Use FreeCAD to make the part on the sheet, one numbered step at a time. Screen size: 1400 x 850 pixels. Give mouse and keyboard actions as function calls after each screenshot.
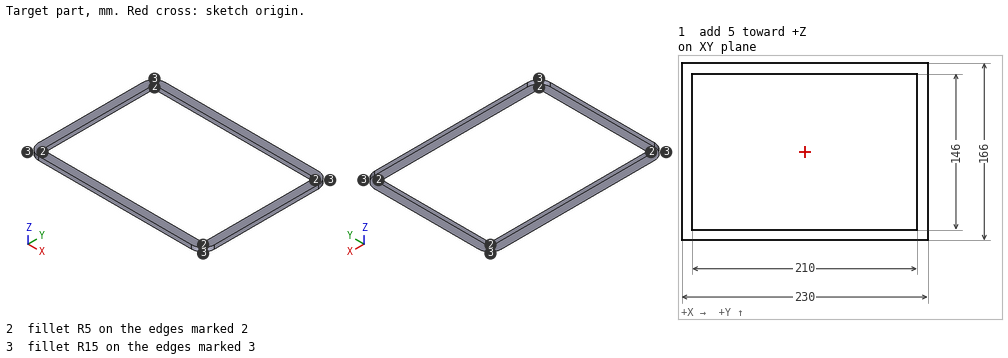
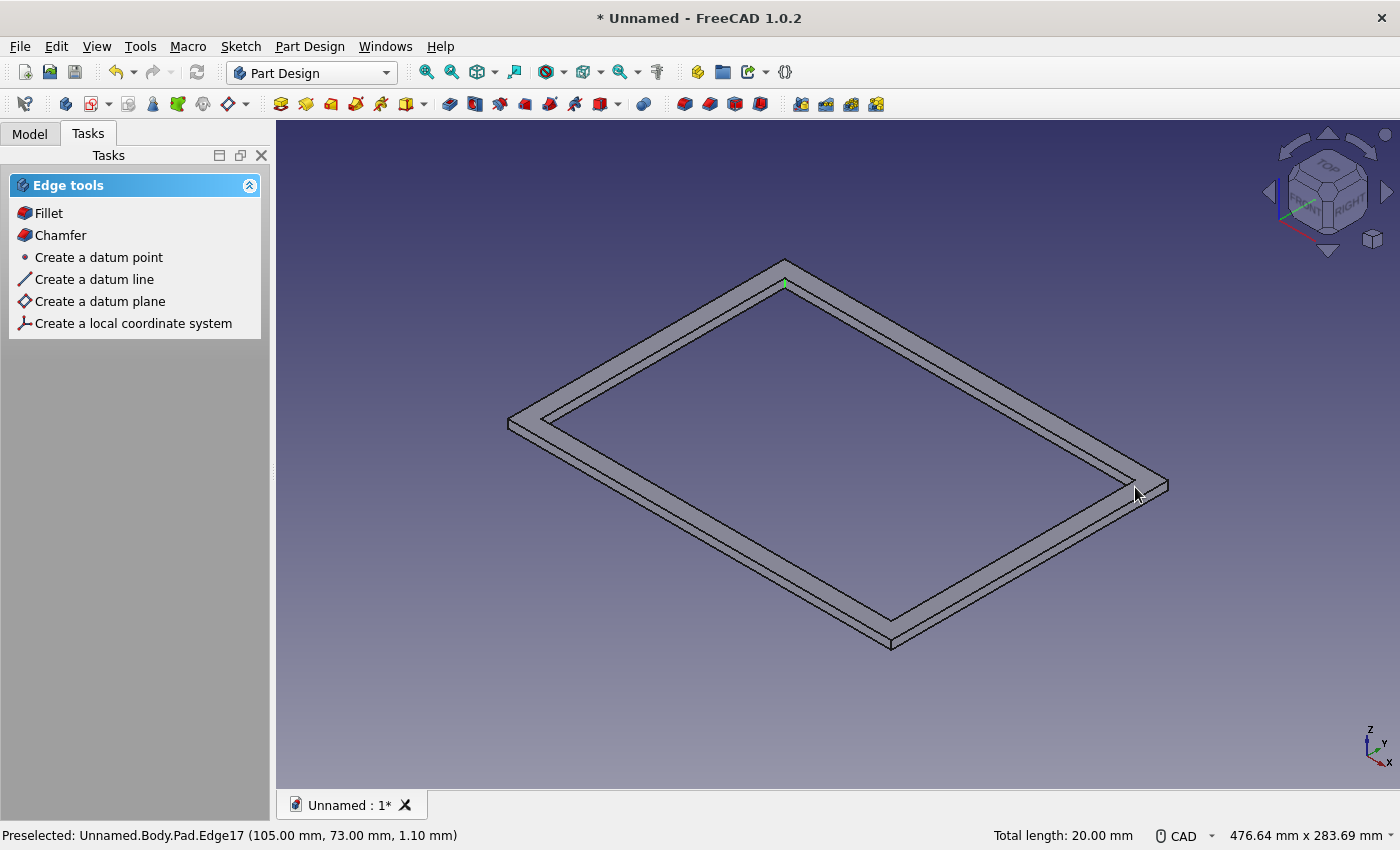
click(685, 104)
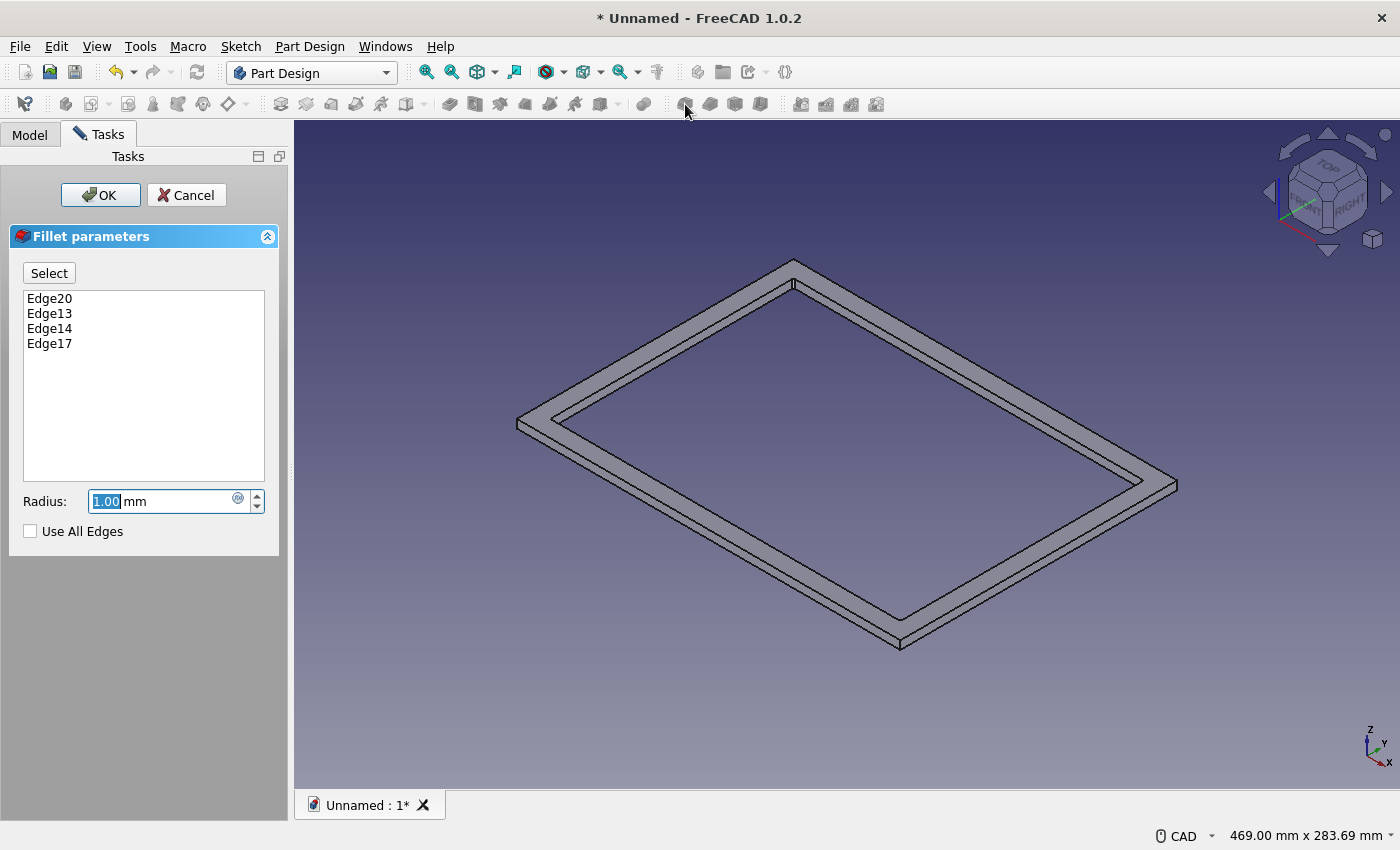
text(5)
key(Tab)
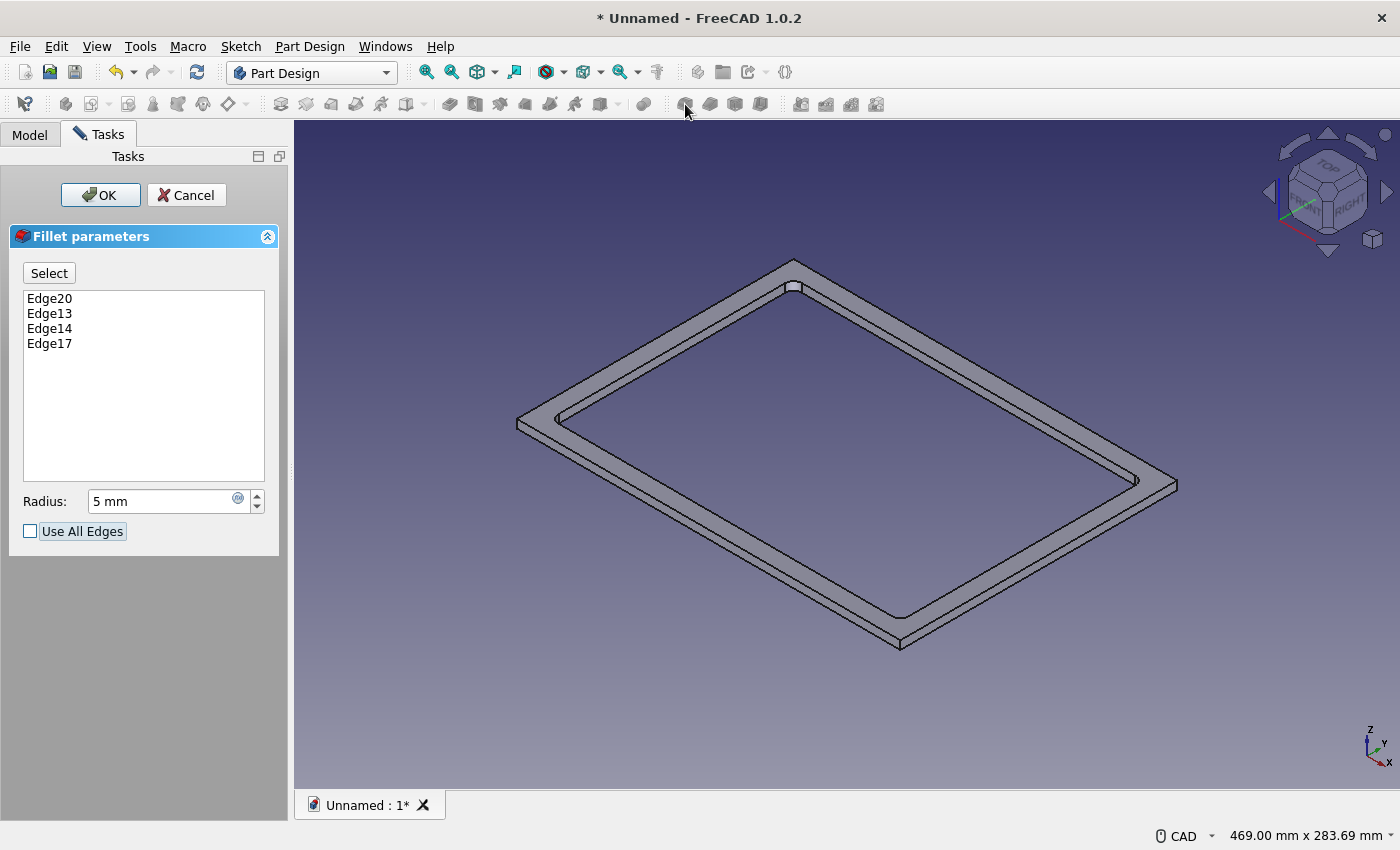
click(101, 195)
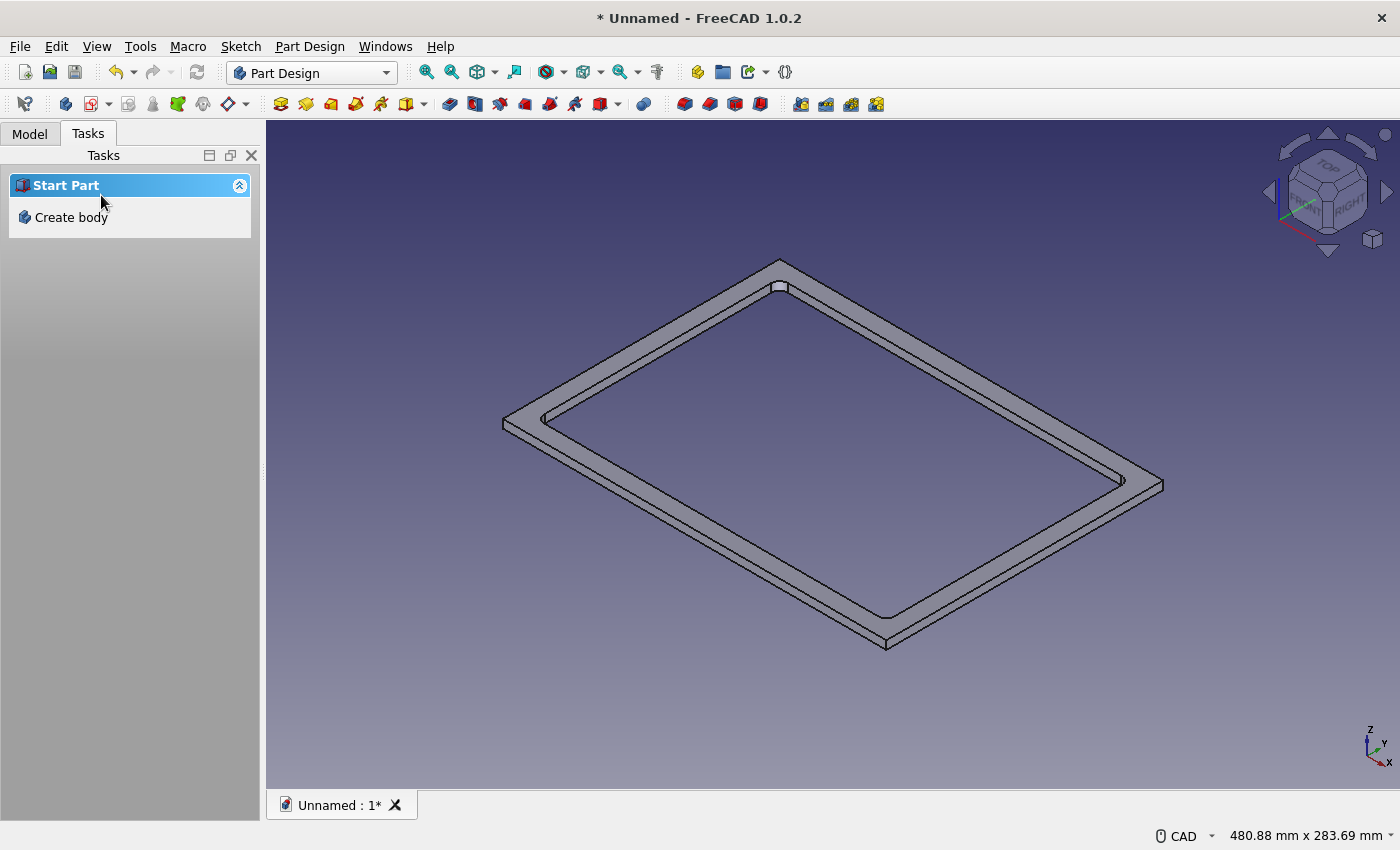
click(886, 646)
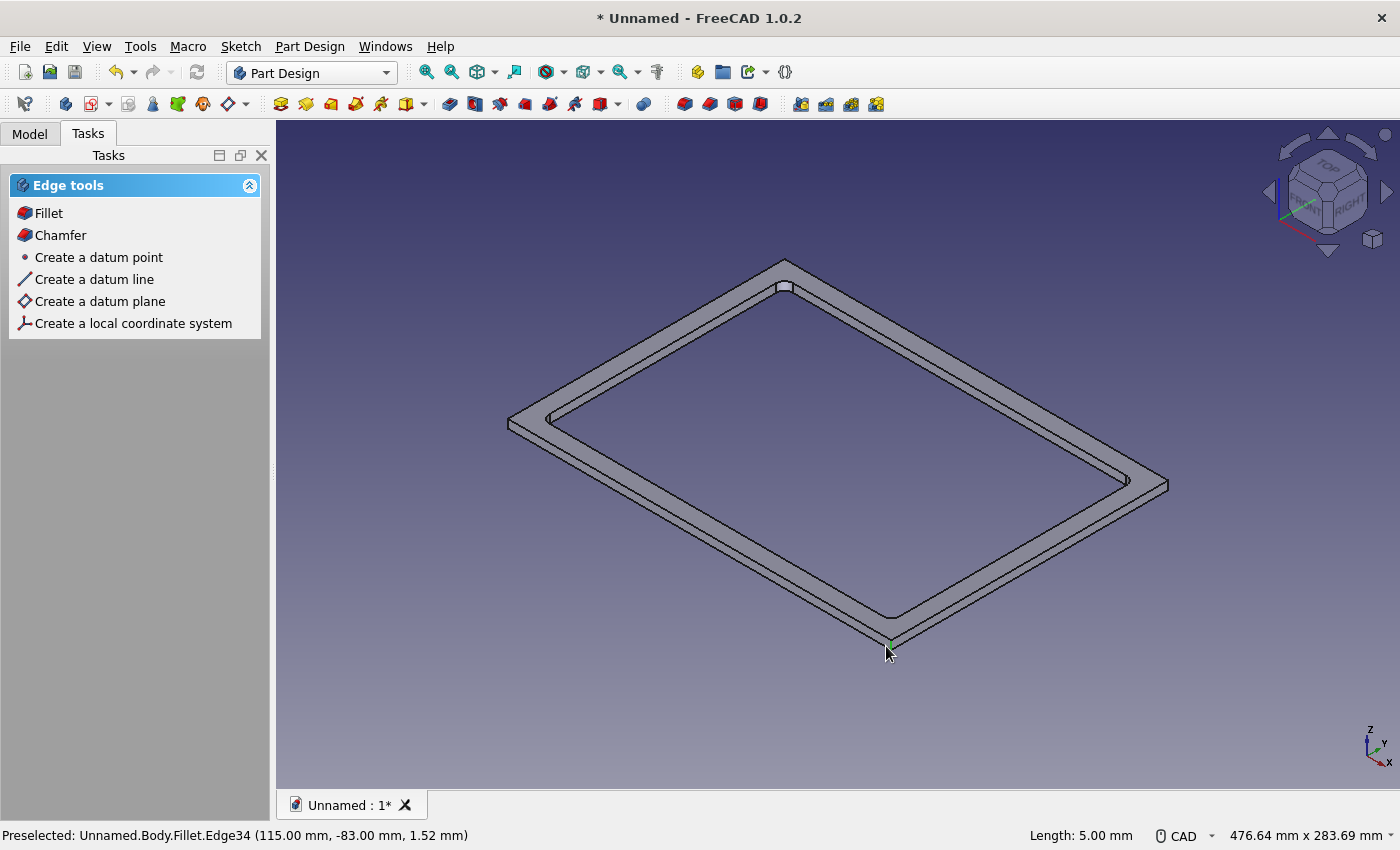
scroll(785, 263, up, 7)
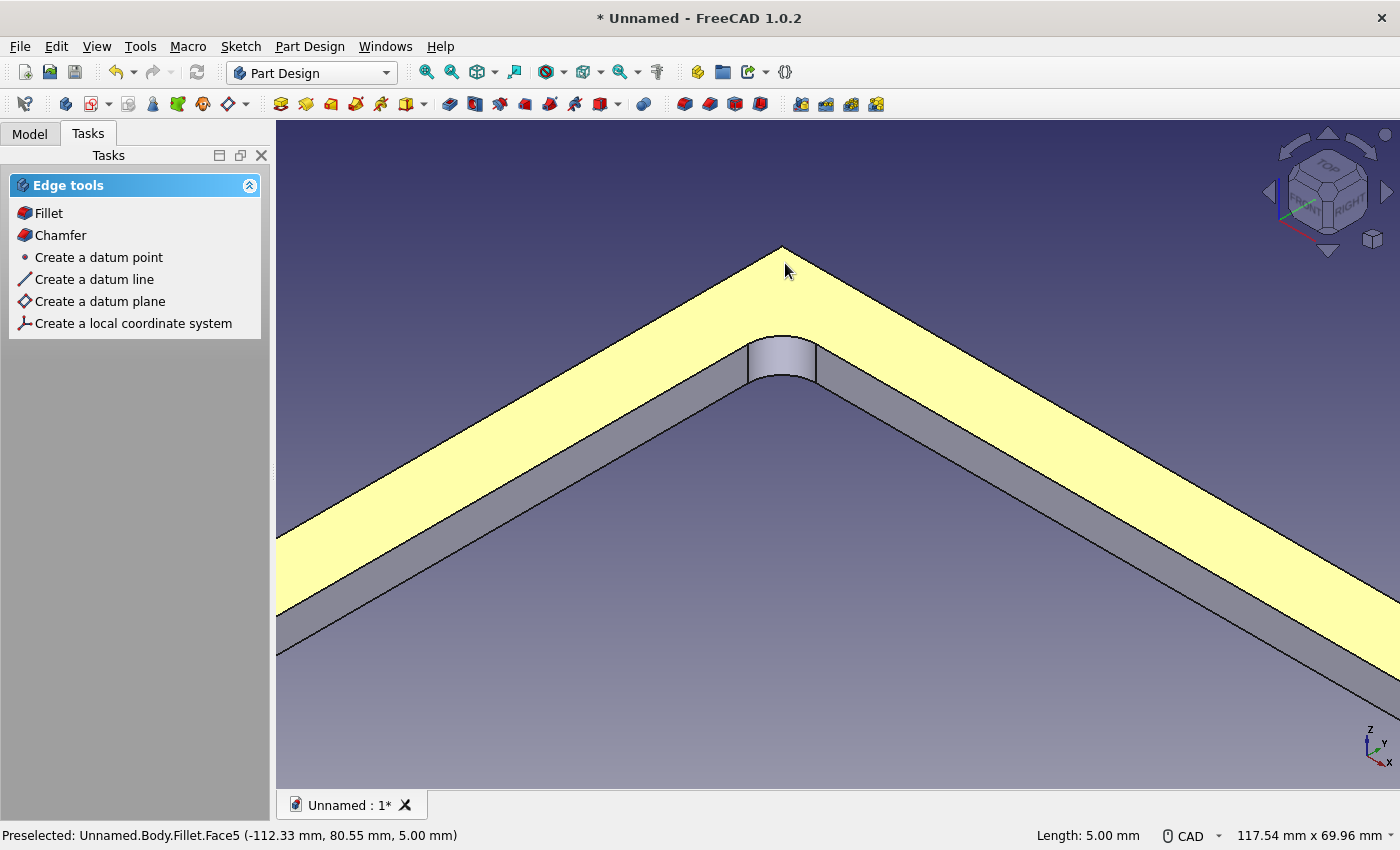
key(v)
key(f)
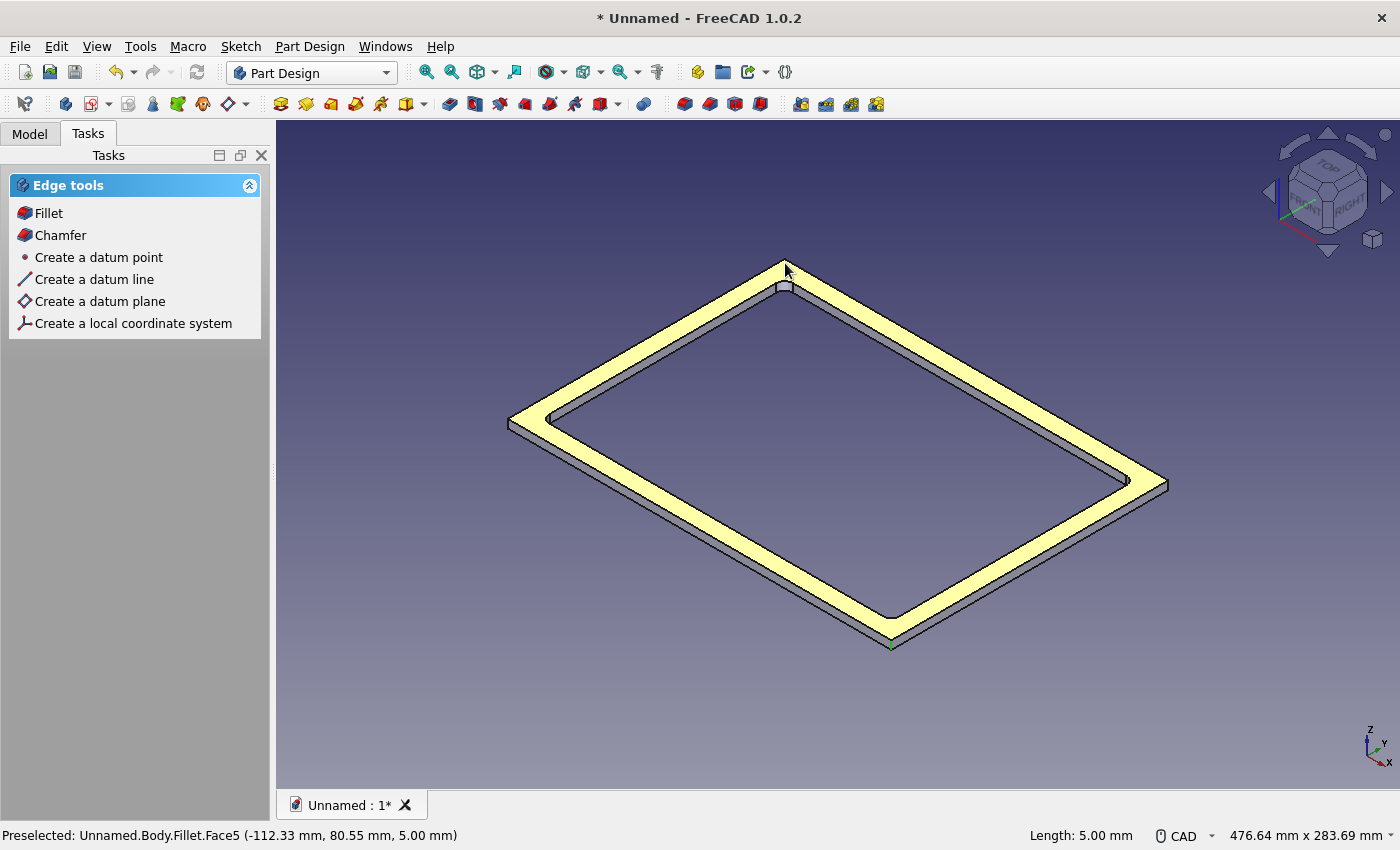
key(2)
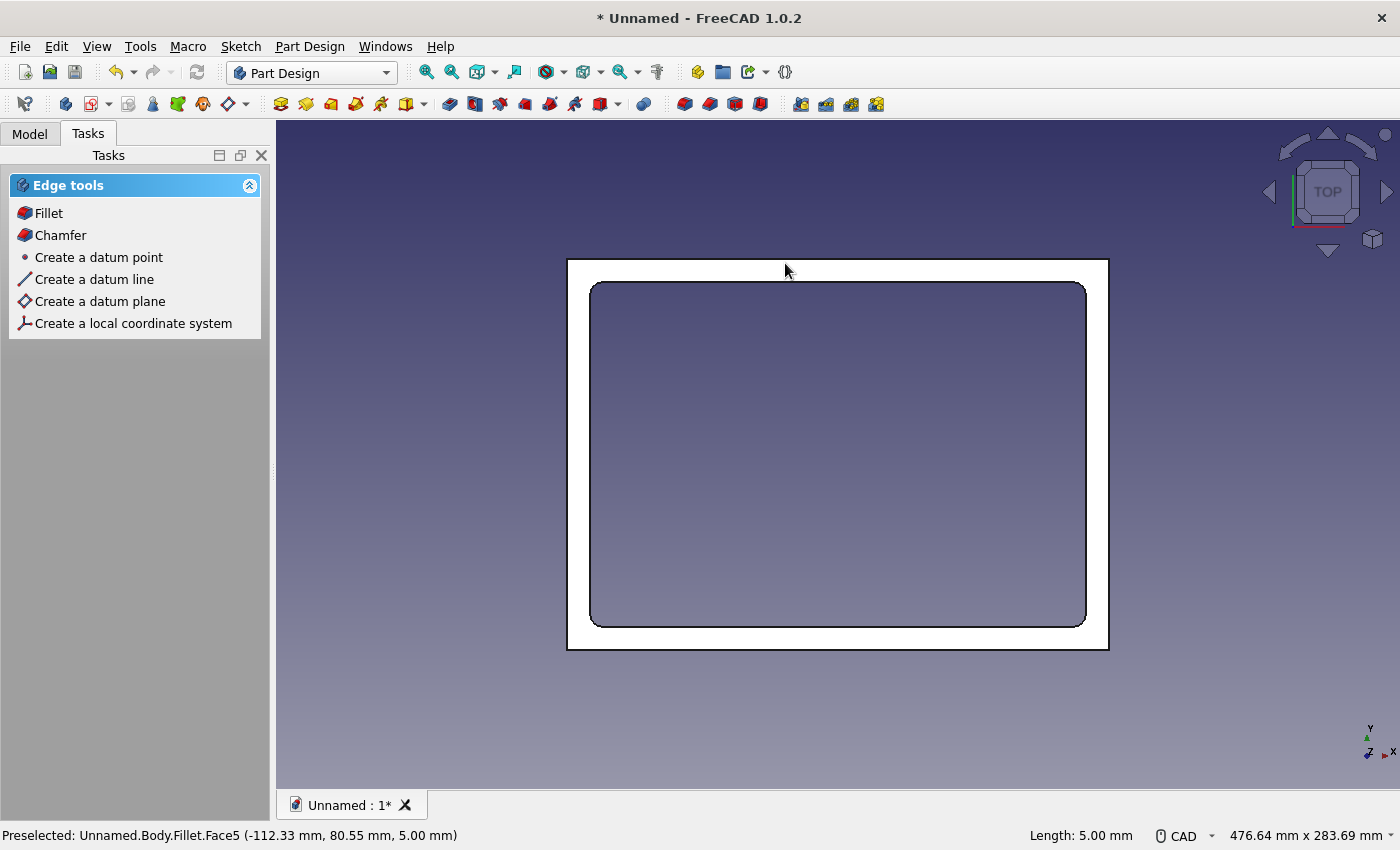
scroll(567, 258, up, 7)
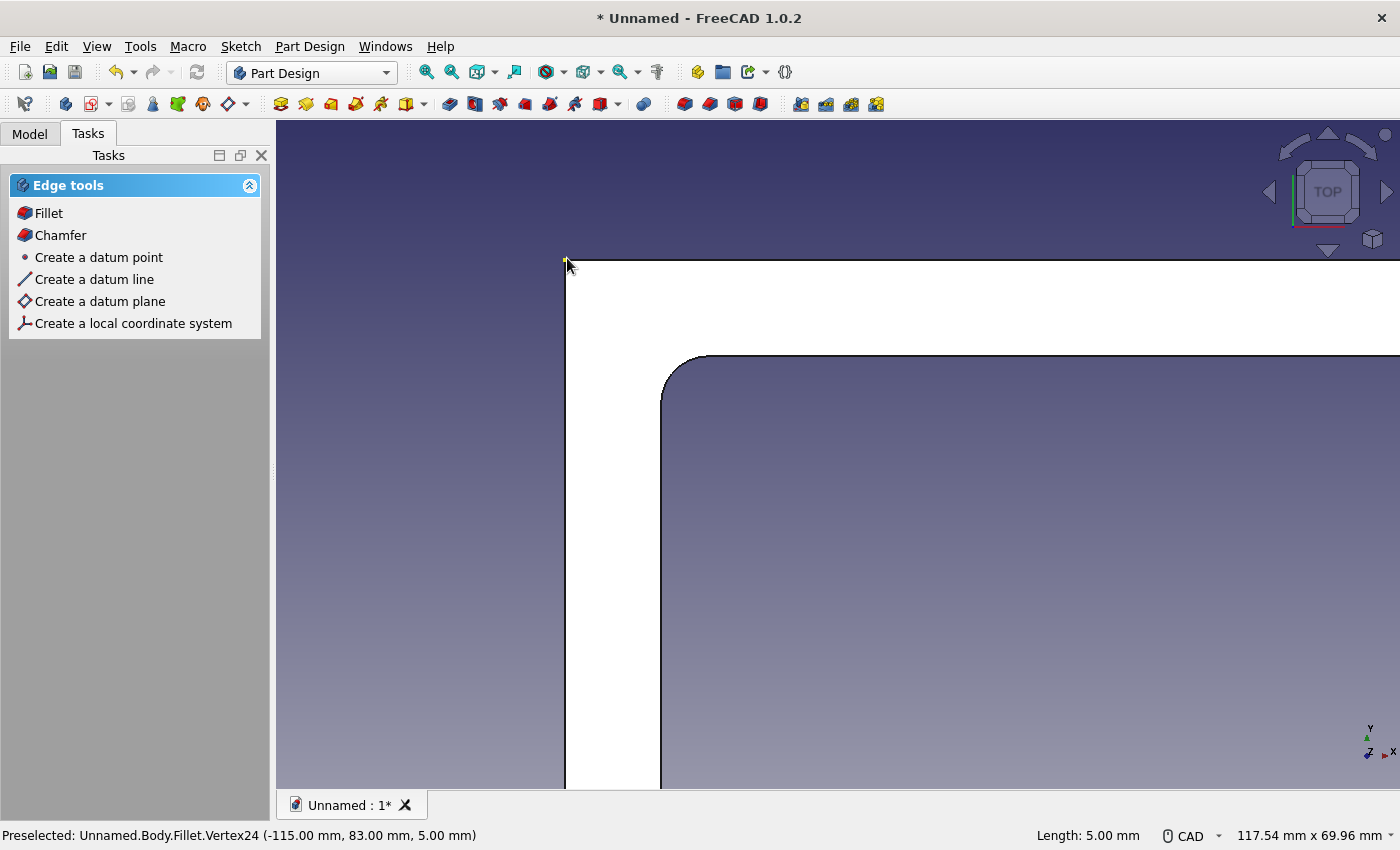
key(v)
key(f)